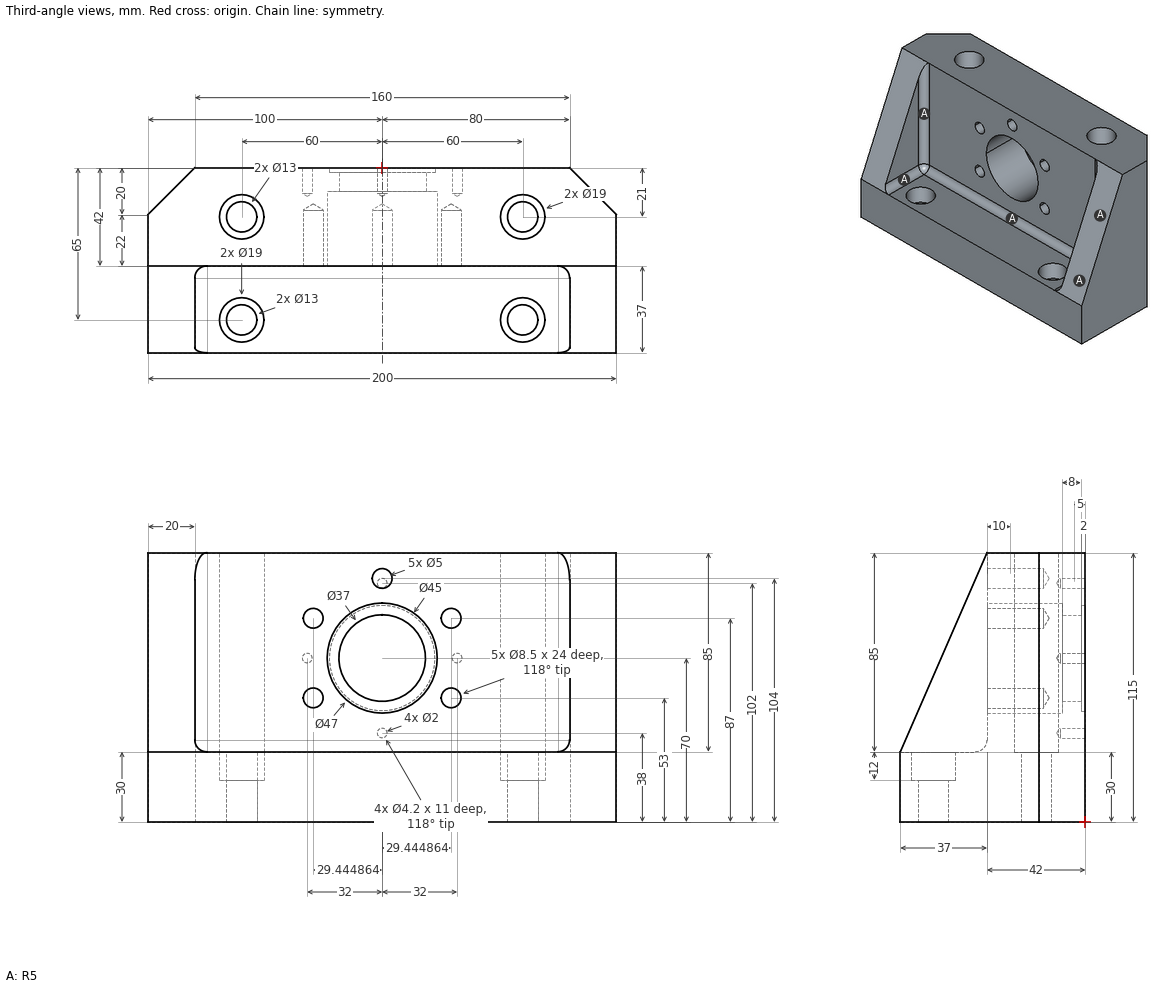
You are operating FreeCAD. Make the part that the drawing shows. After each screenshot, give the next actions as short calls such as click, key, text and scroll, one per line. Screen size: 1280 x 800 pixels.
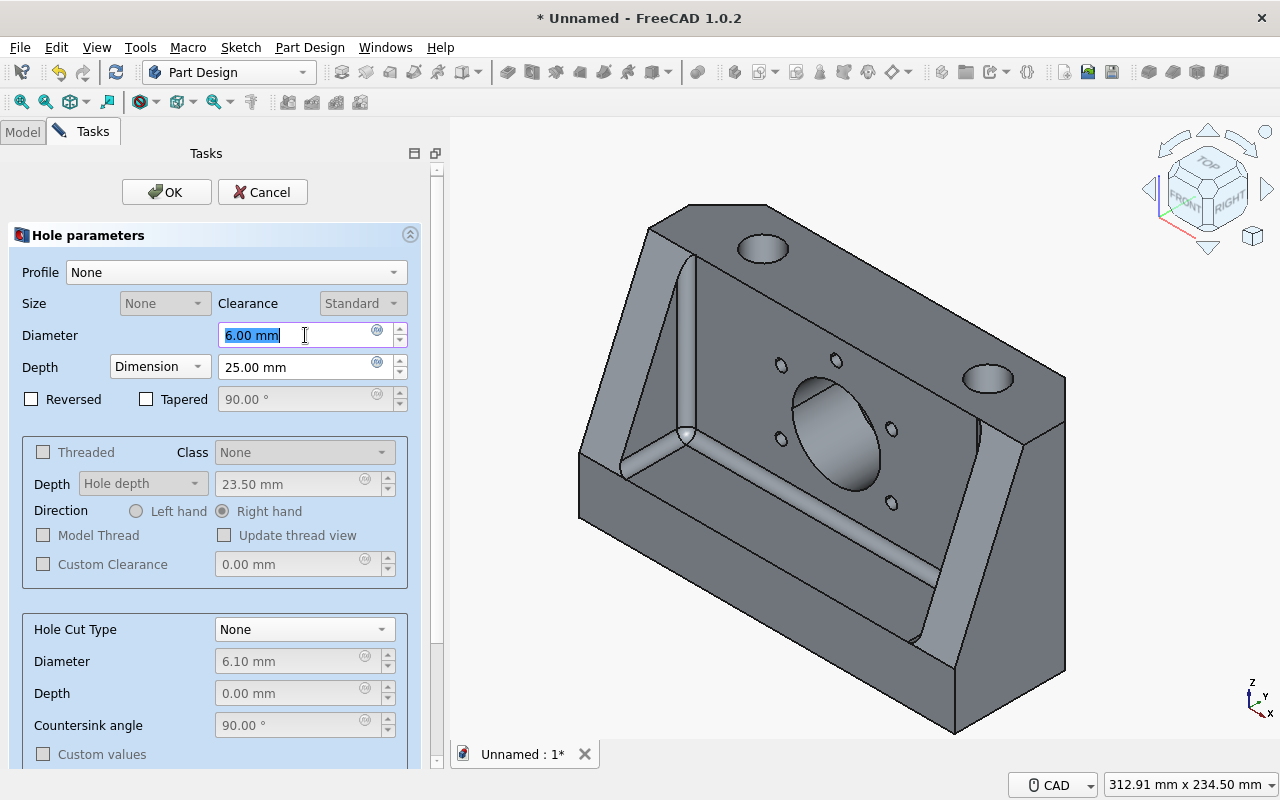
text(8.5)
key(Tab)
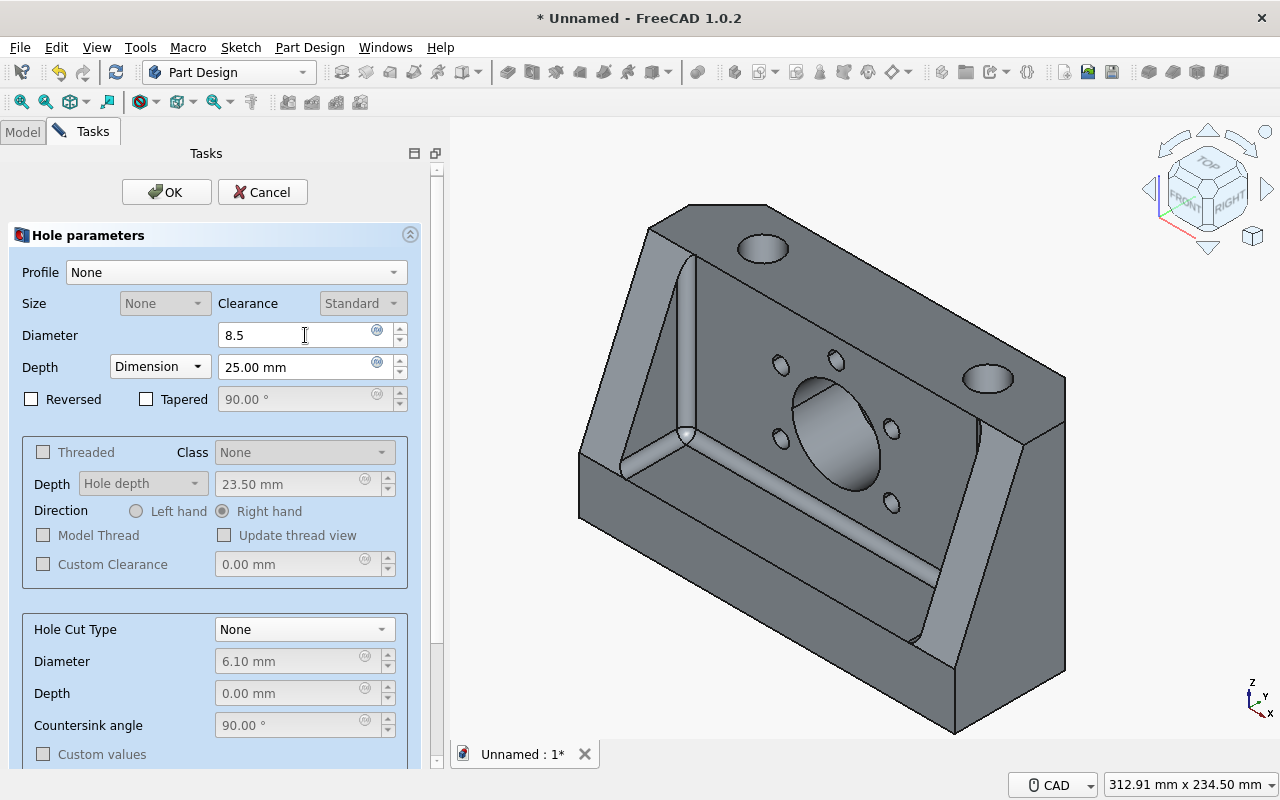
triple_click(305, 367)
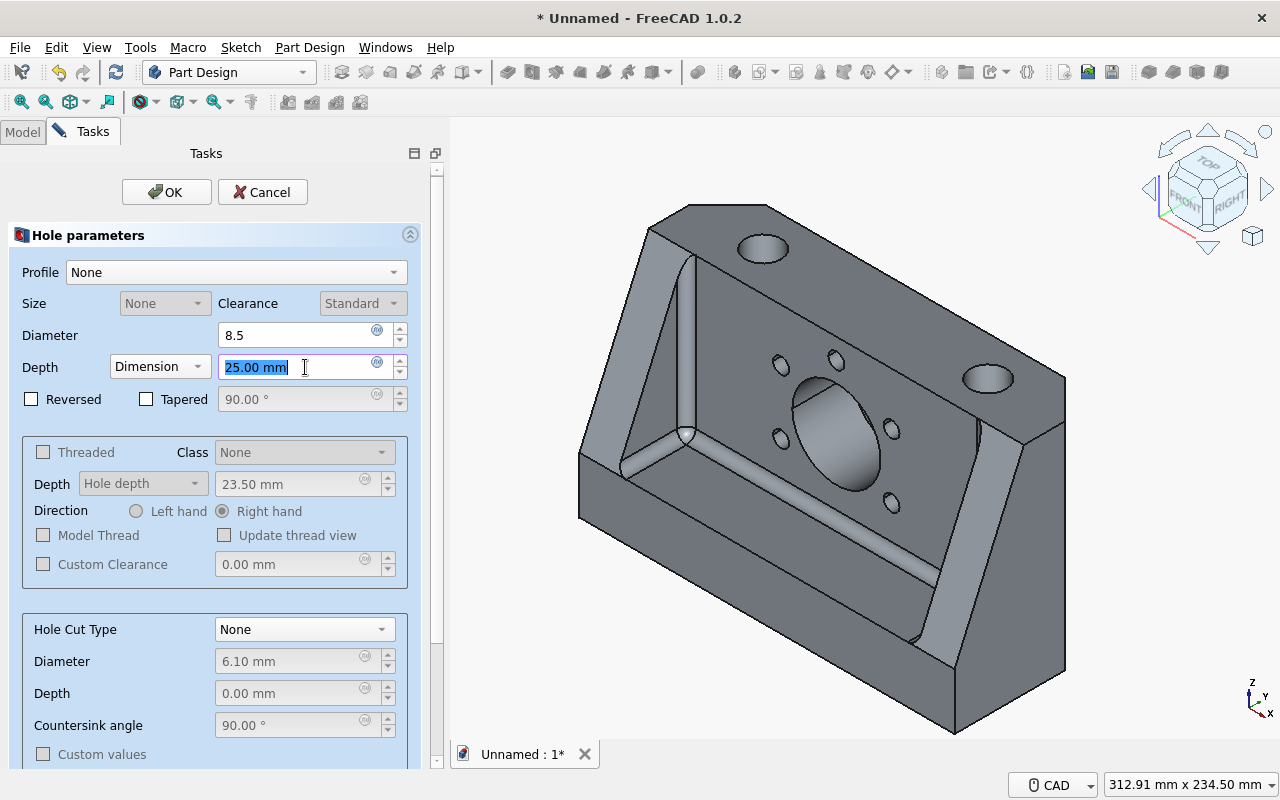
text(24)
key(Tab)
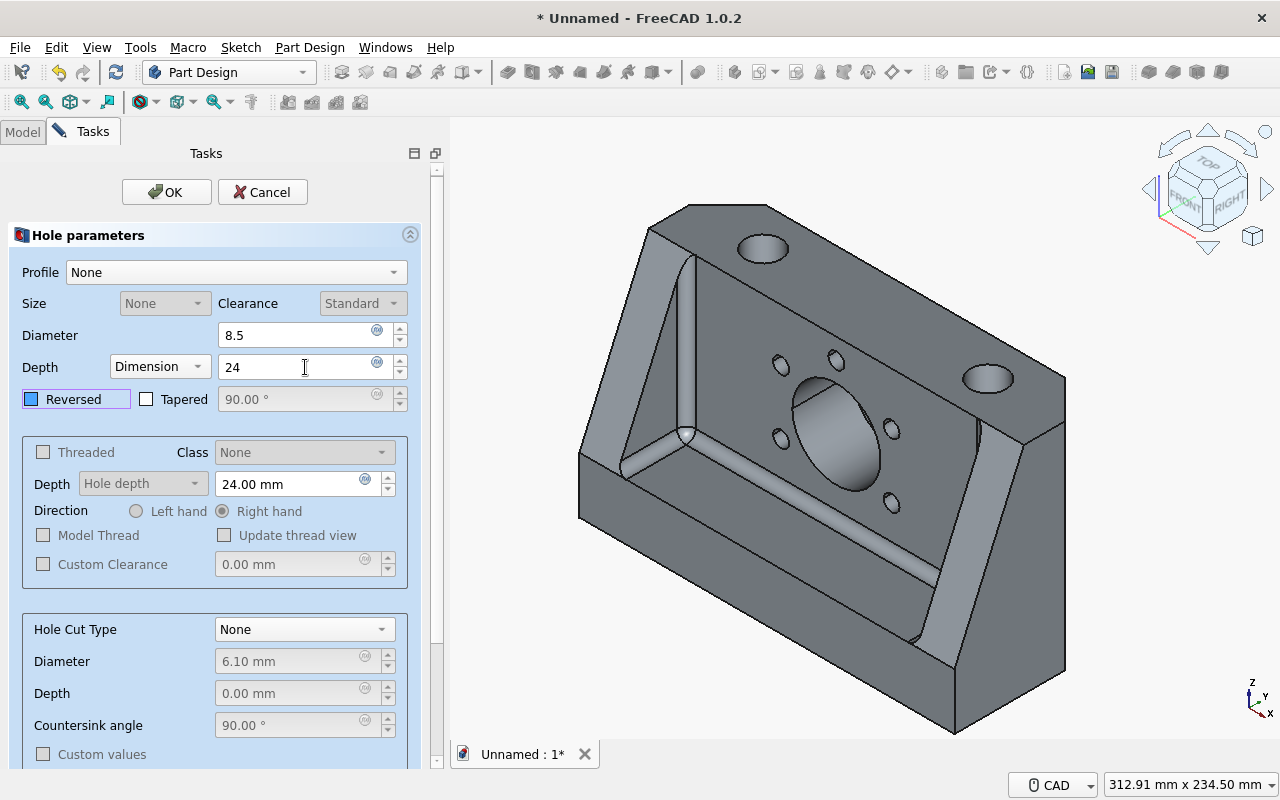
click(167, 192)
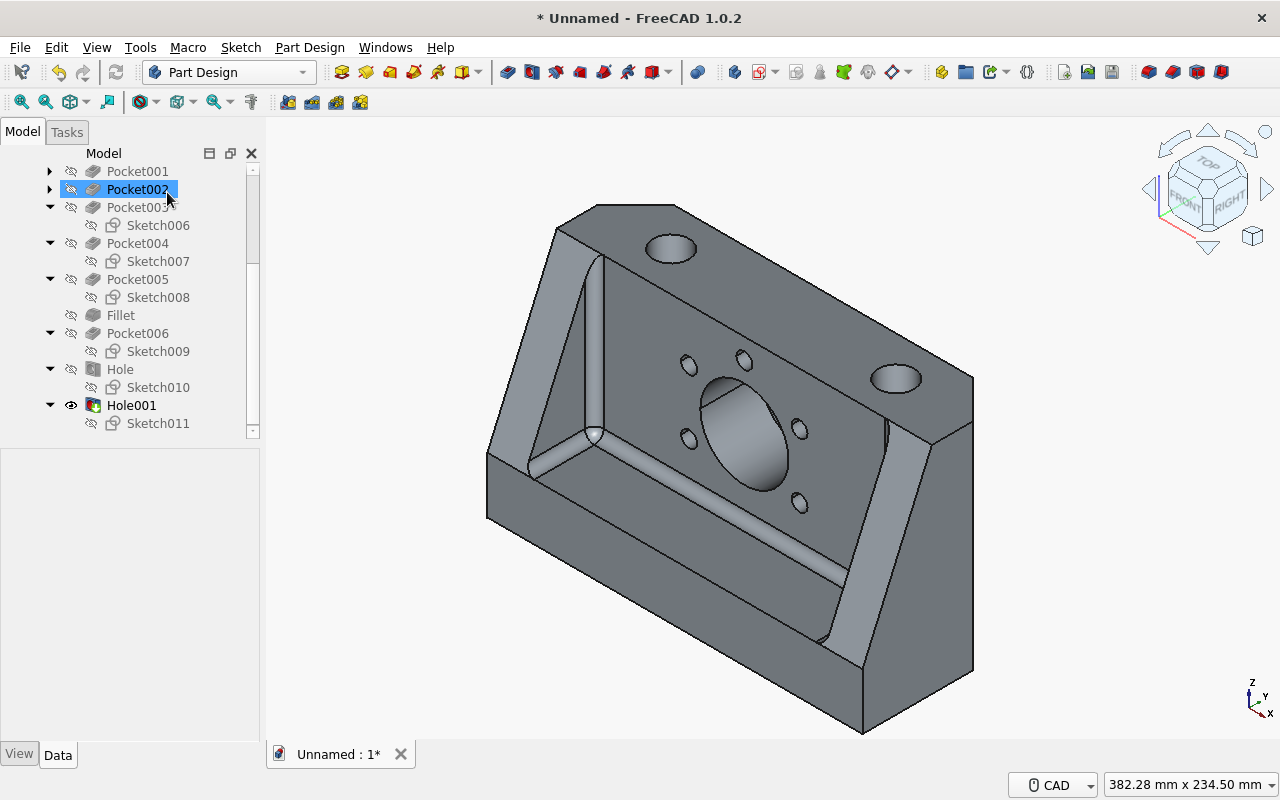
click(785, 589)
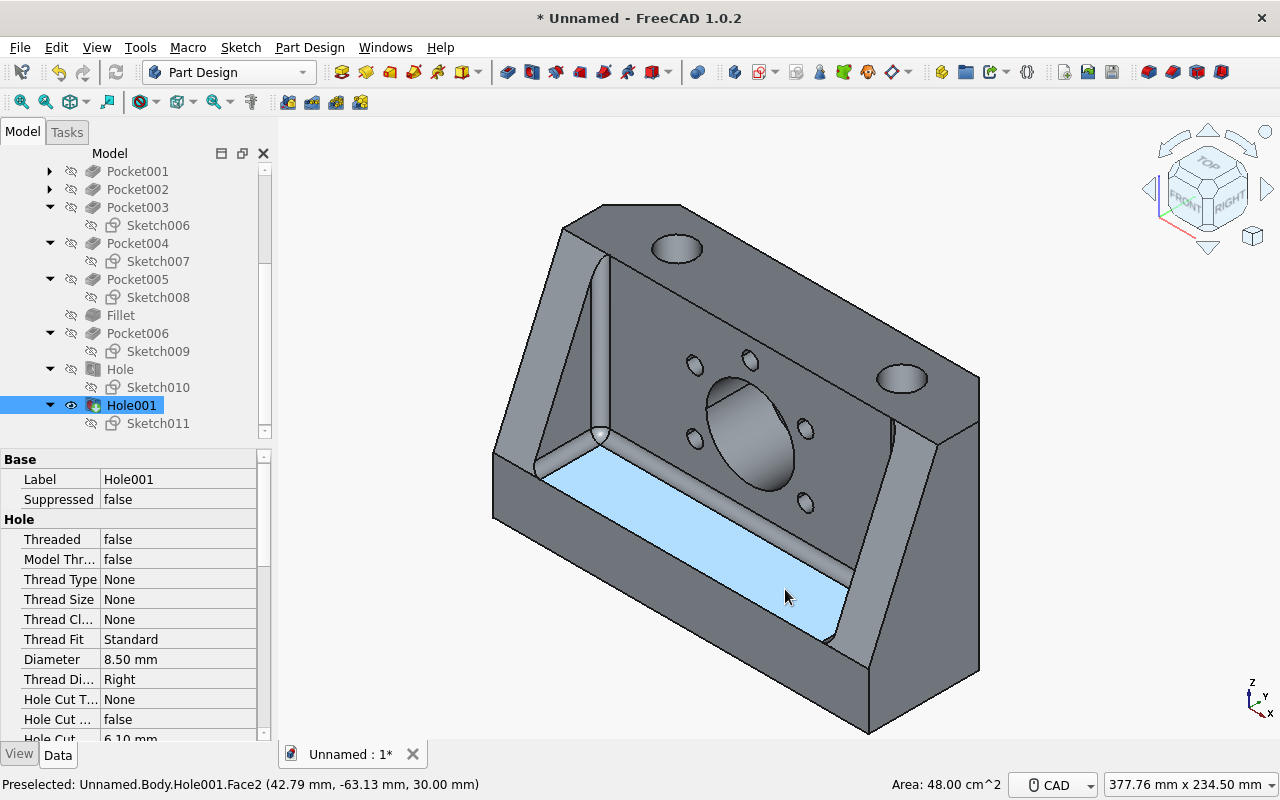
click(760, 72)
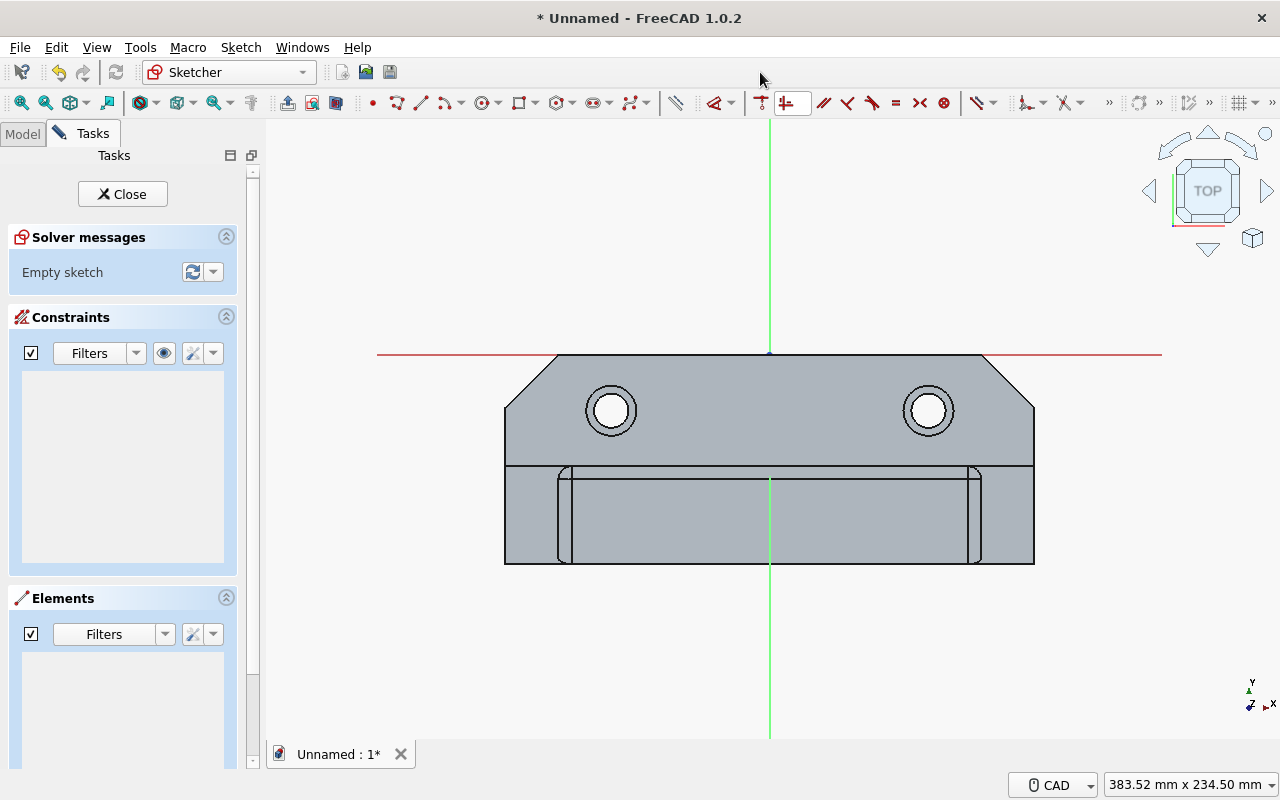
scroll(903, 492, up, 2)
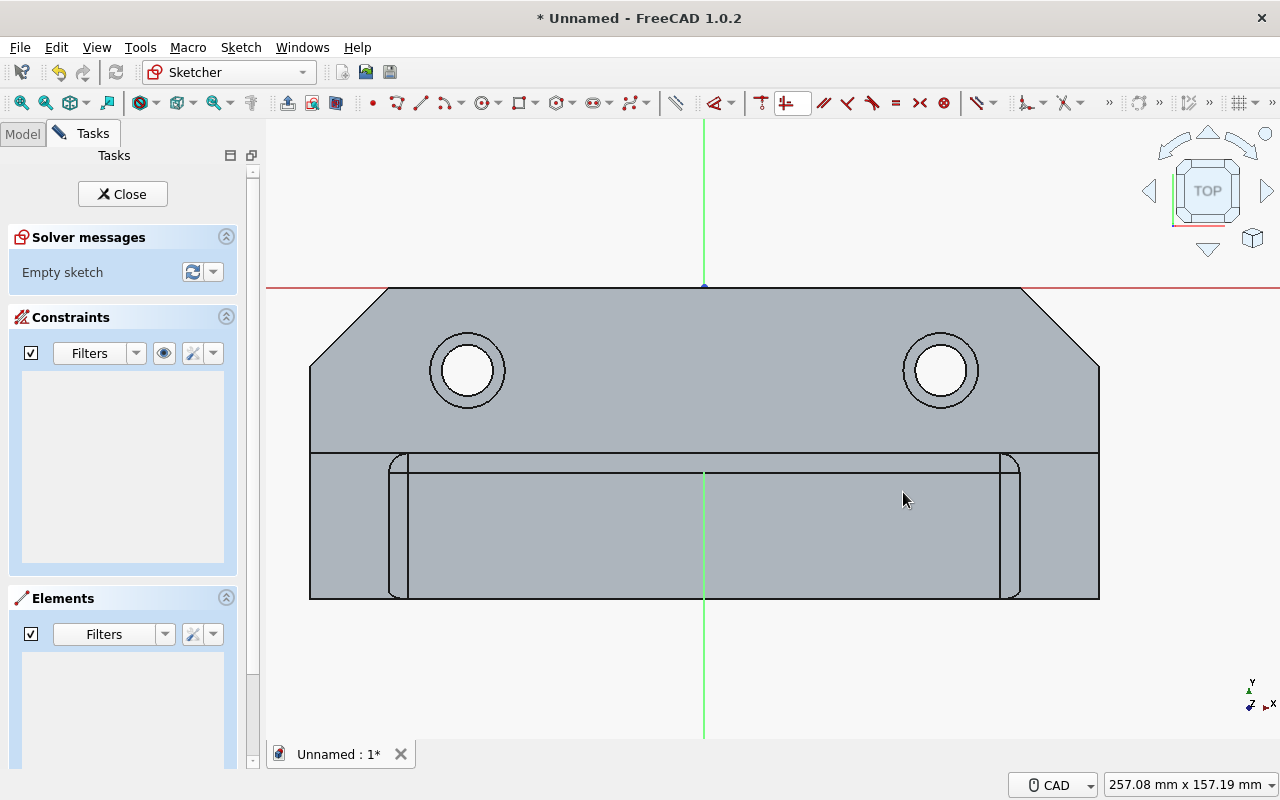
click(482, 104)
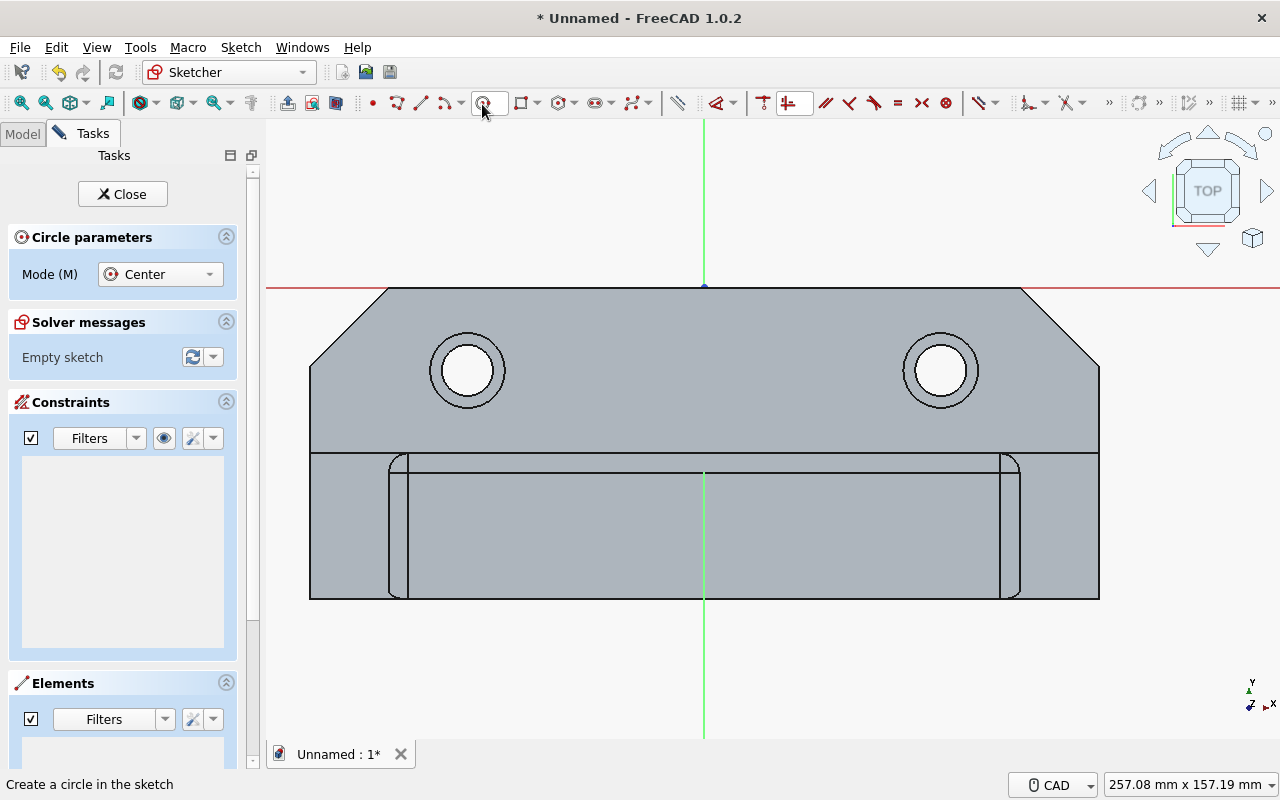
click(467, 544)
move(486, 526)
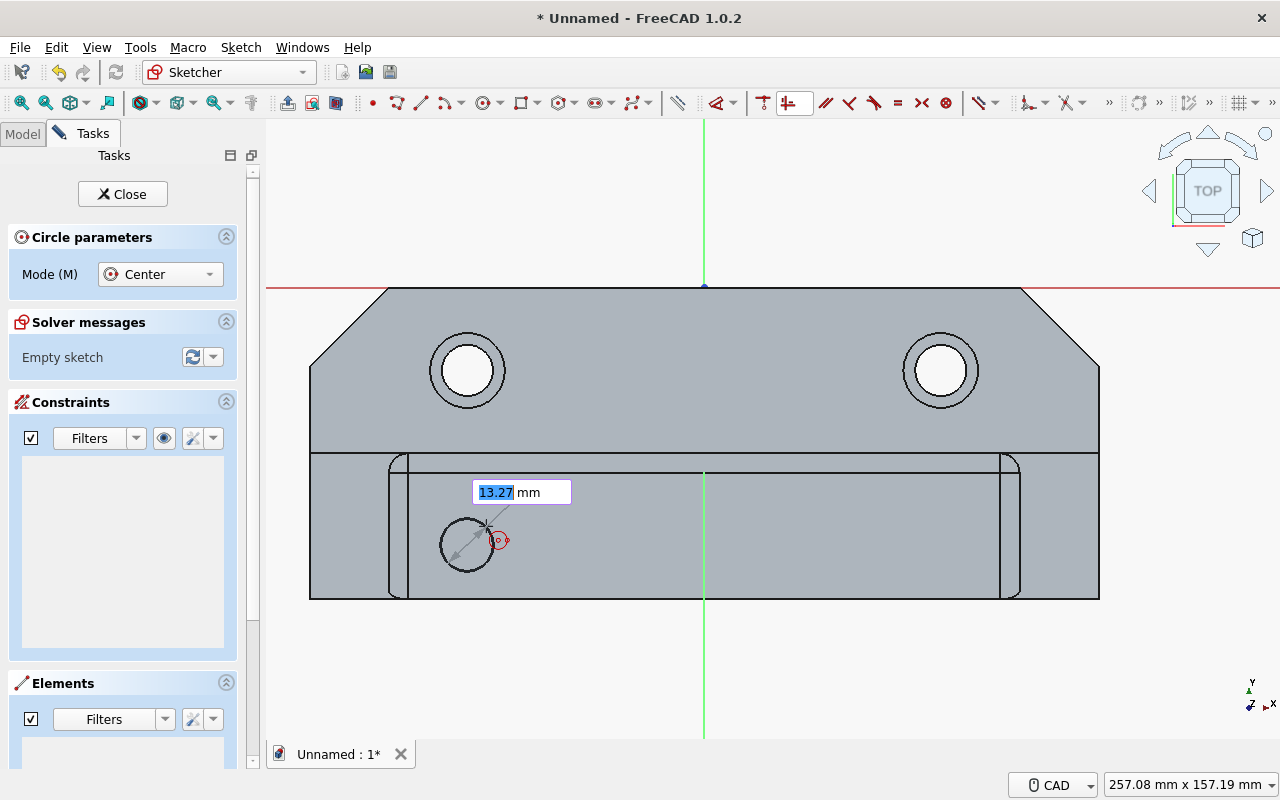
text(13)
key(Return)